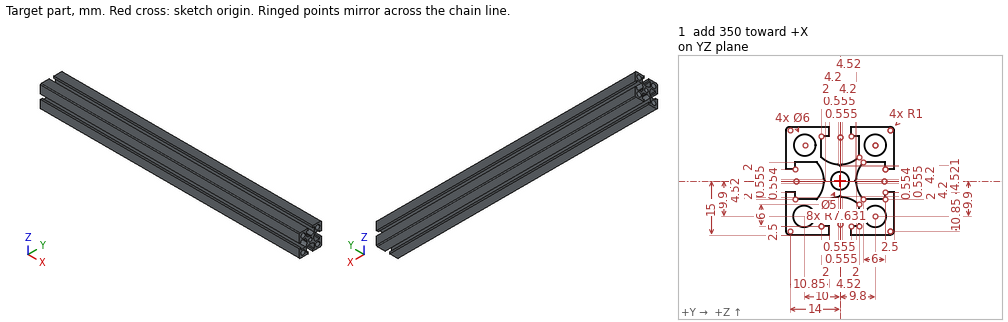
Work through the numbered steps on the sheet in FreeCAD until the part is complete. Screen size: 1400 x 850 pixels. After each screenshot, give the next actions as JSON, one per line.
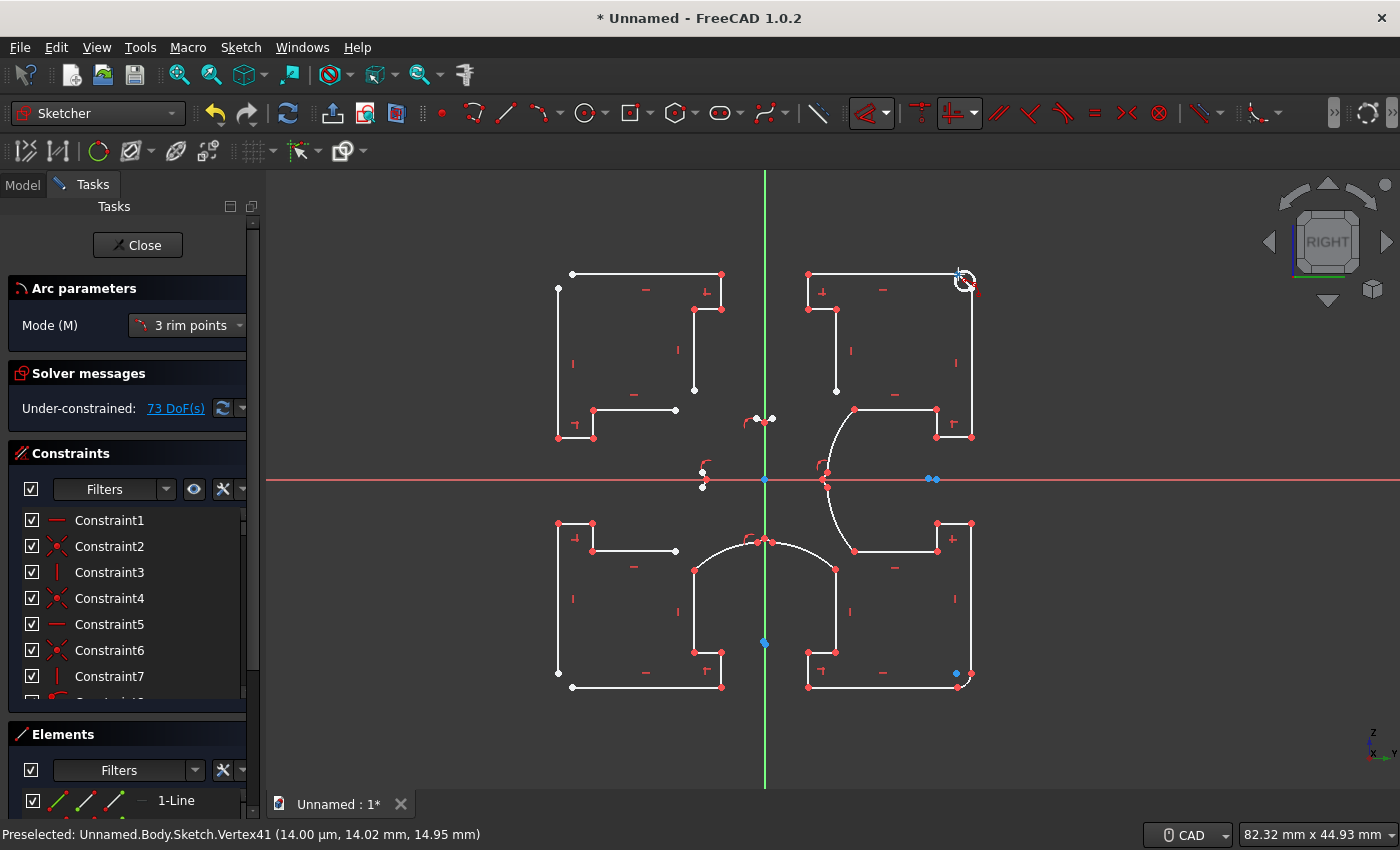
{"action": "scroll", "coordinate": [967, 277], "scroll_direction": "up", "scroll_amount": 7}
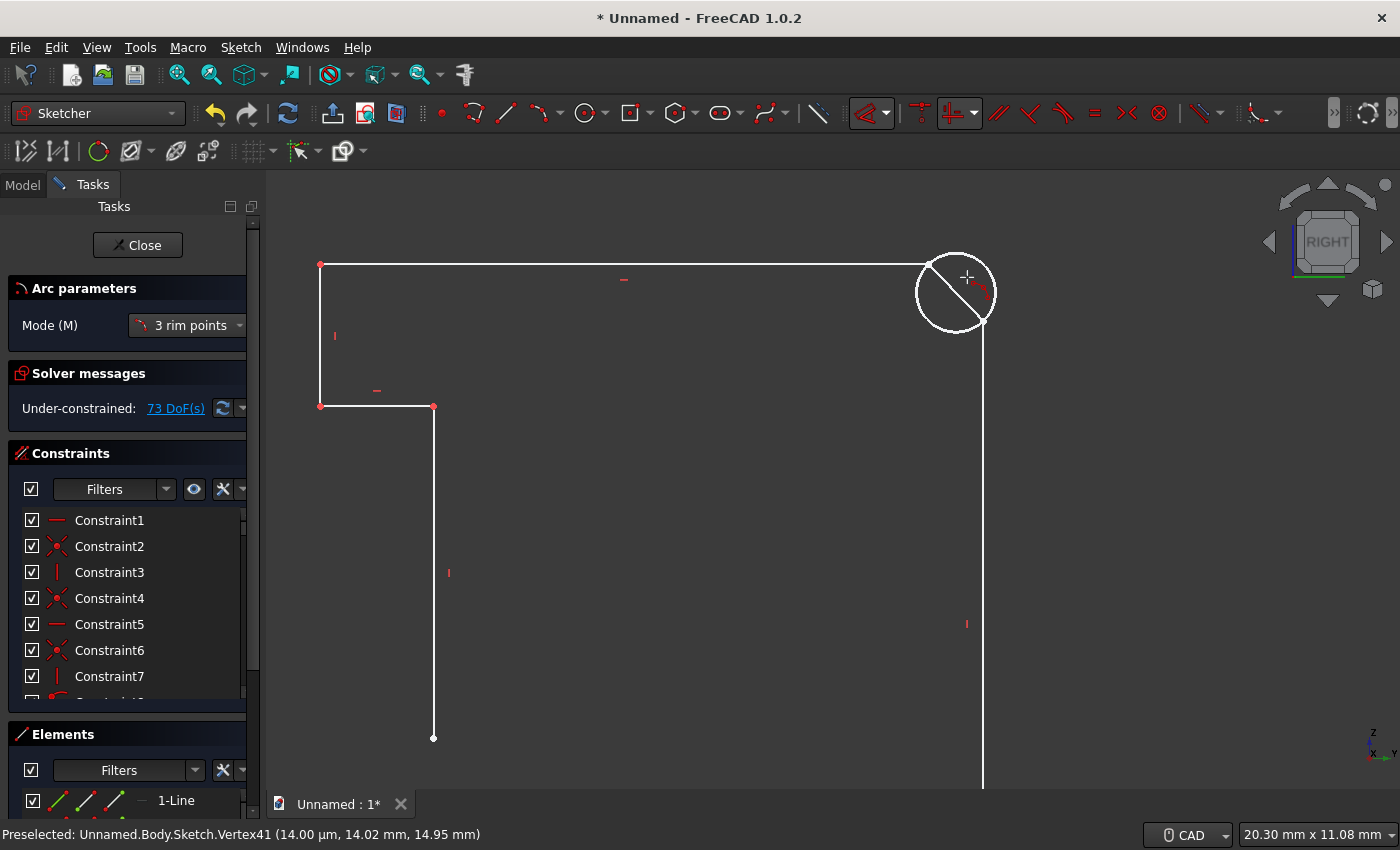
{"action": "left_click", "coordinate": [967, 278]}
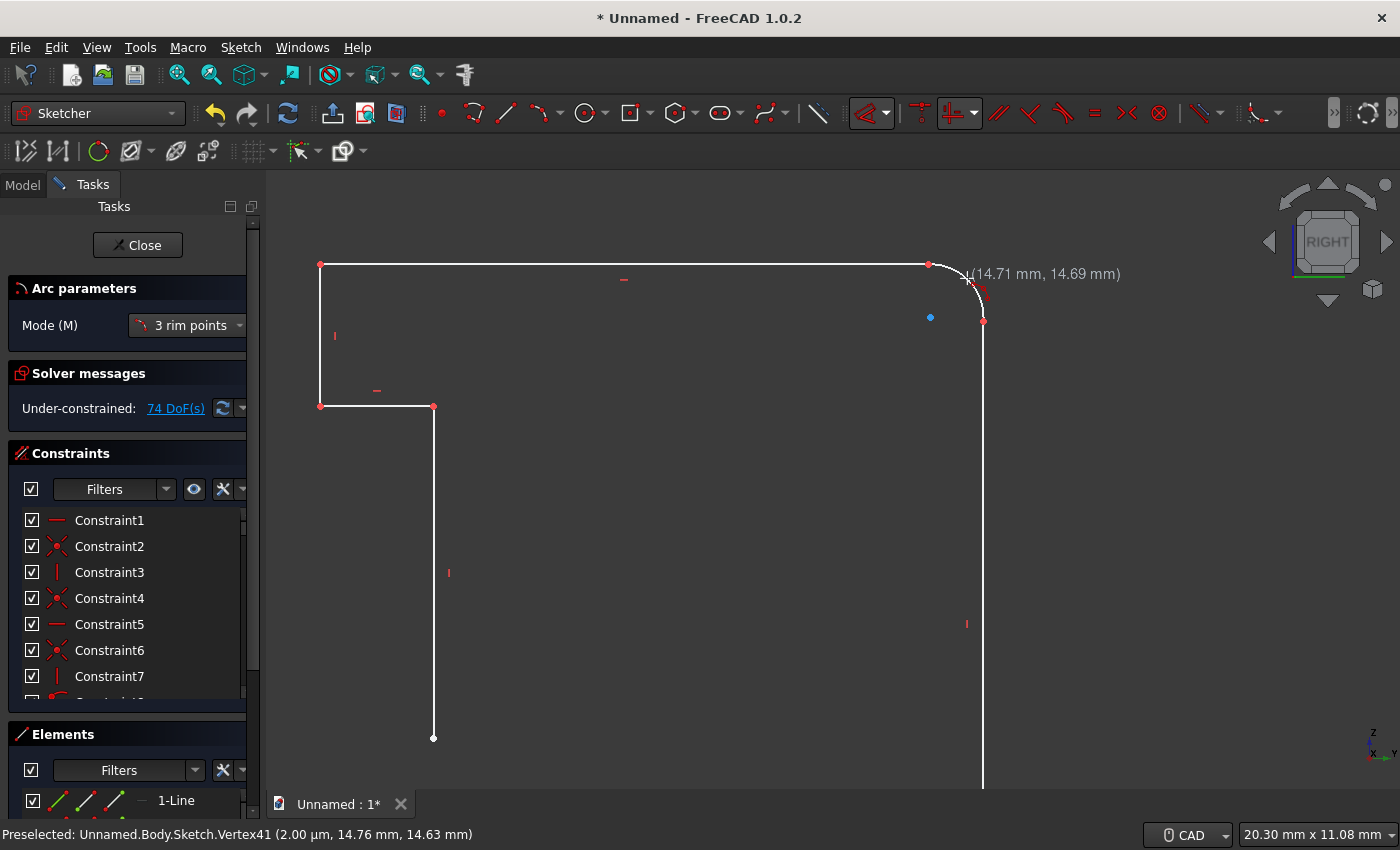
{"action": "scroll", "coordinate": [967, 277], "scroll_direction": "down", "scroll_amount": 7}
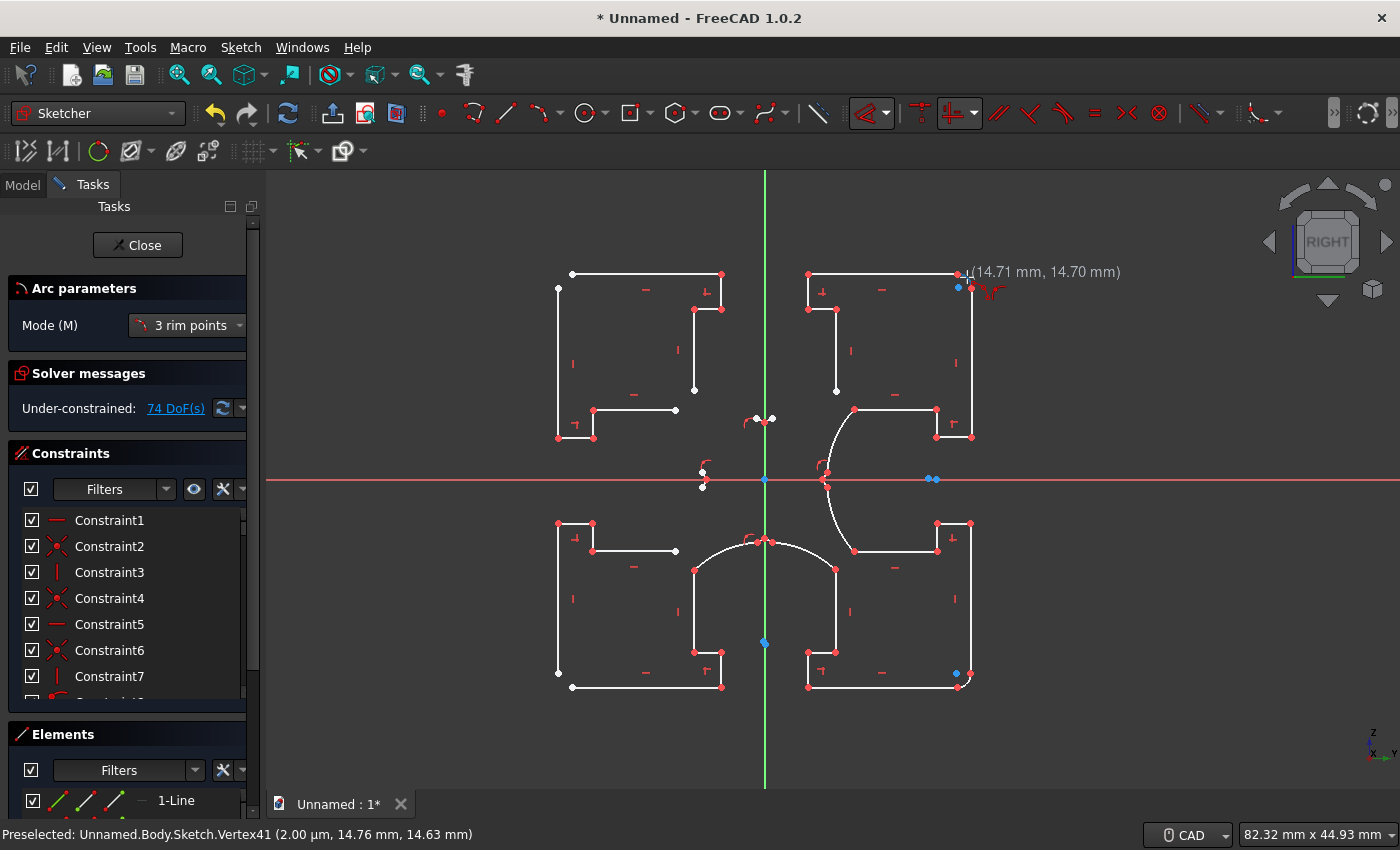
{"action": "left_click", "coordinate": [836, 391]}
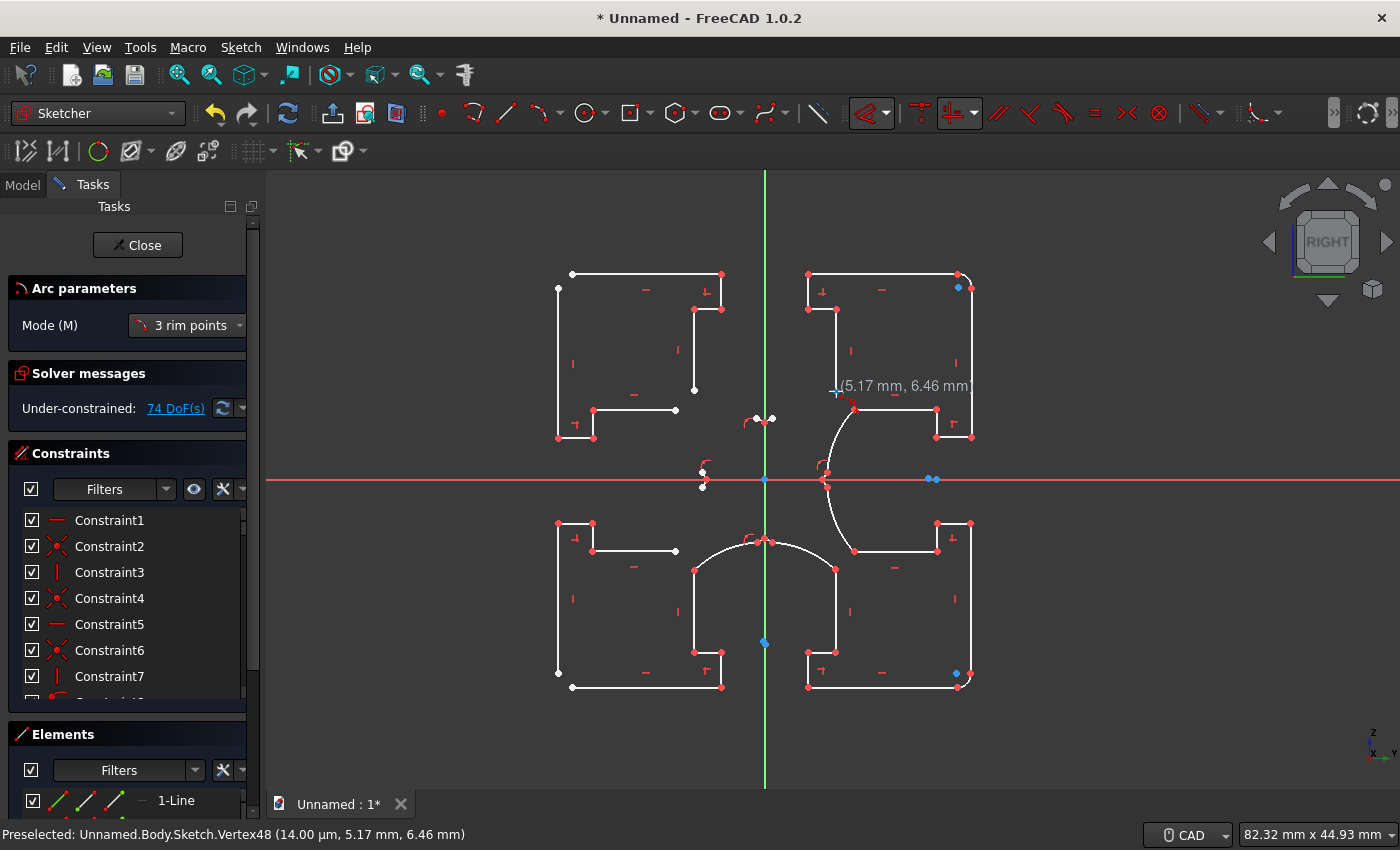
{"action": "scroll", "coordinate": [772, 418], "scroll_direction": "up", "scroll_amount": 7}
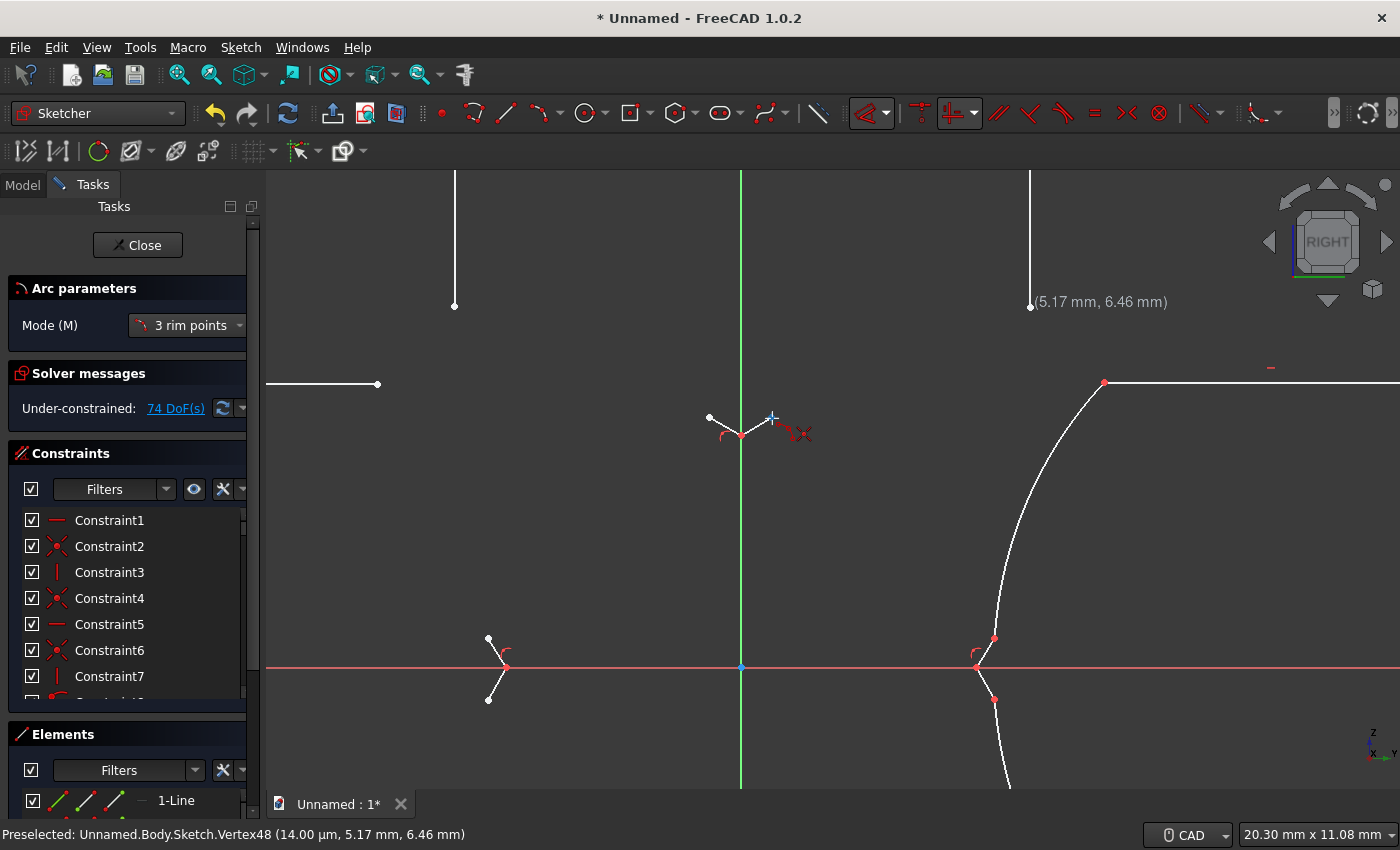
{"action": "left_click", "coordinate": [772, 418]}
{"action": "left_click", "coordinate": [910, 382]}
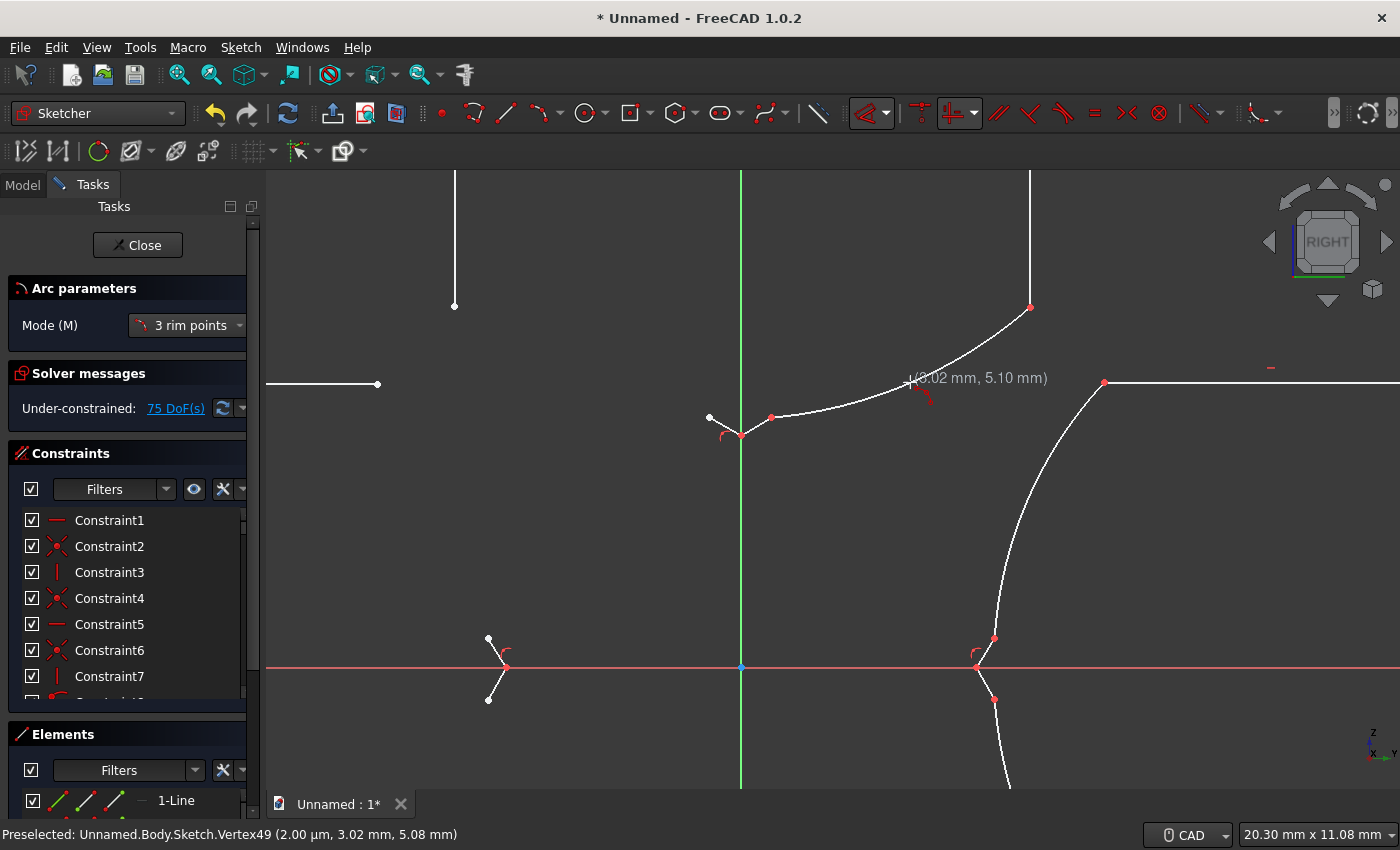
{"action": "left_click", "coordinate": [710, 418]}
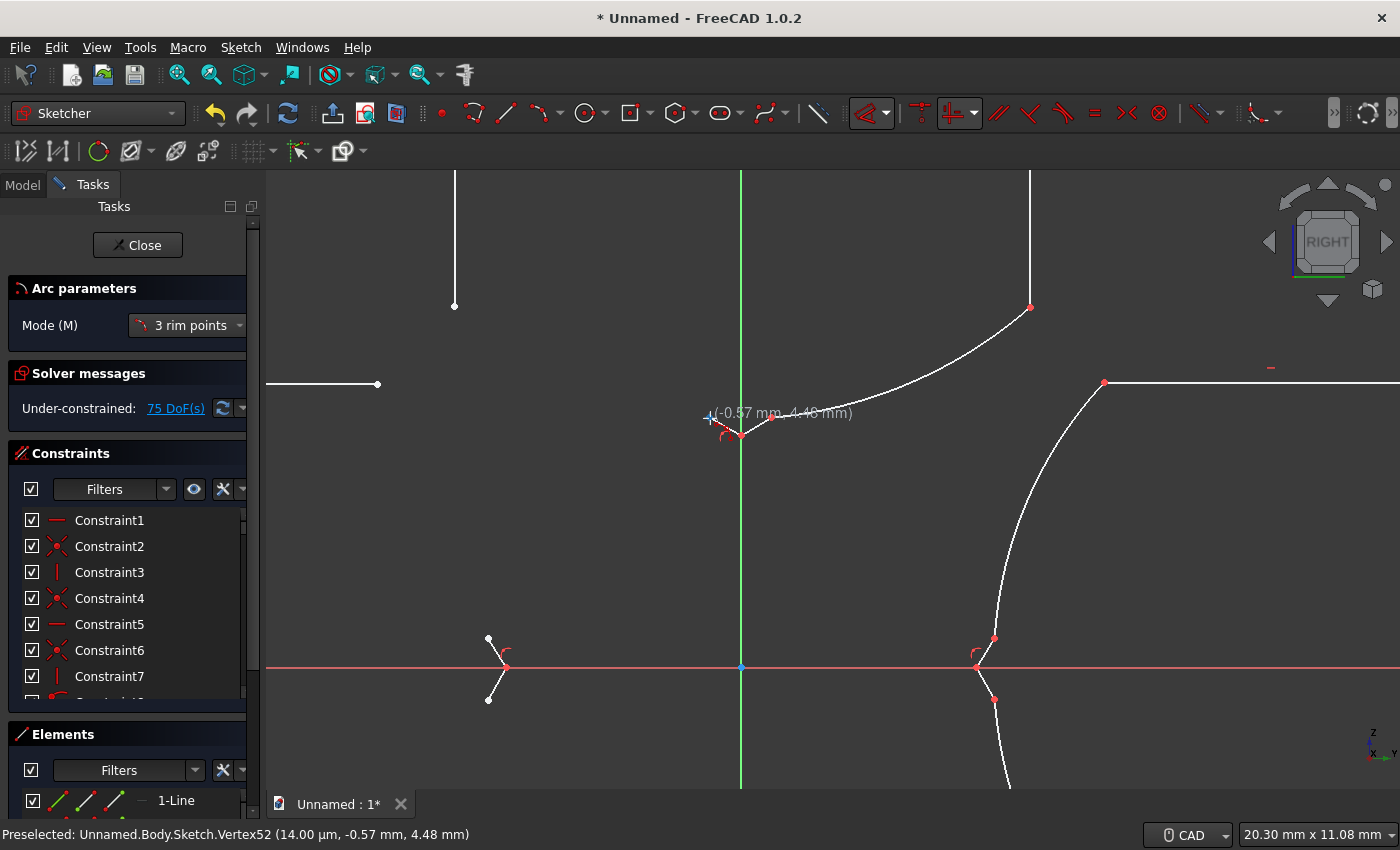
{"action": "scroll", "coordinate": [772, 418], "scroll_direction": "down", "scroll_amount": 7}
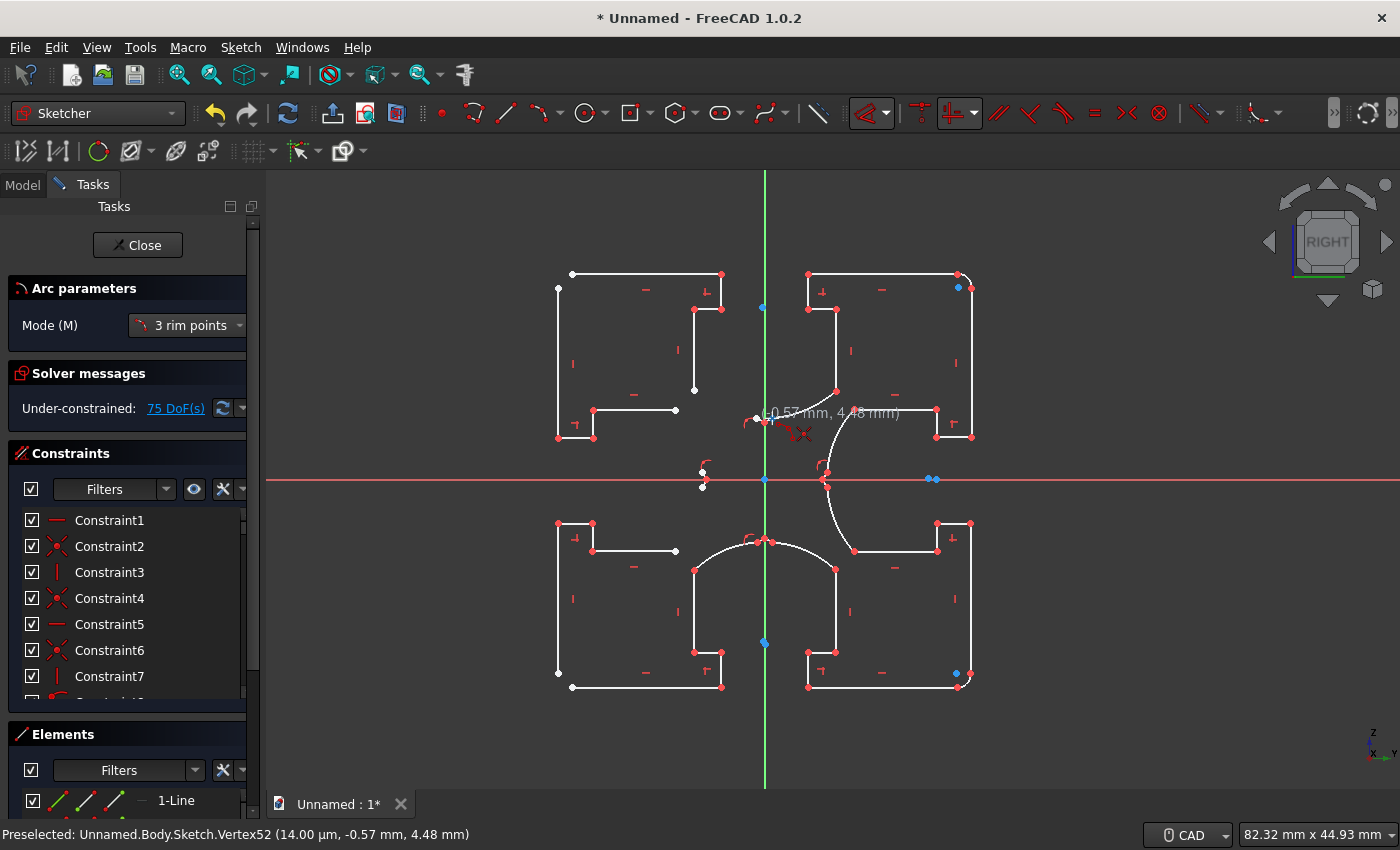
{"action": "left_click", "coordinate": [694, 391]}